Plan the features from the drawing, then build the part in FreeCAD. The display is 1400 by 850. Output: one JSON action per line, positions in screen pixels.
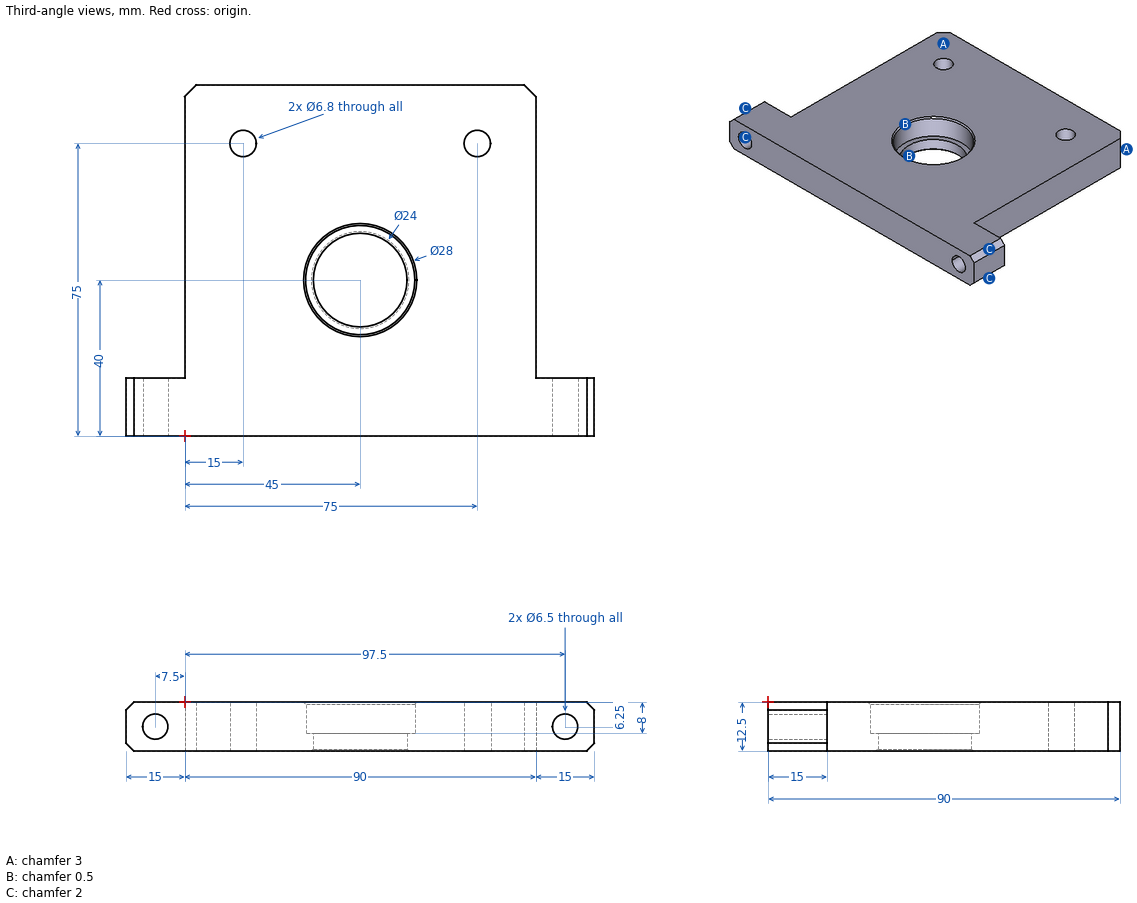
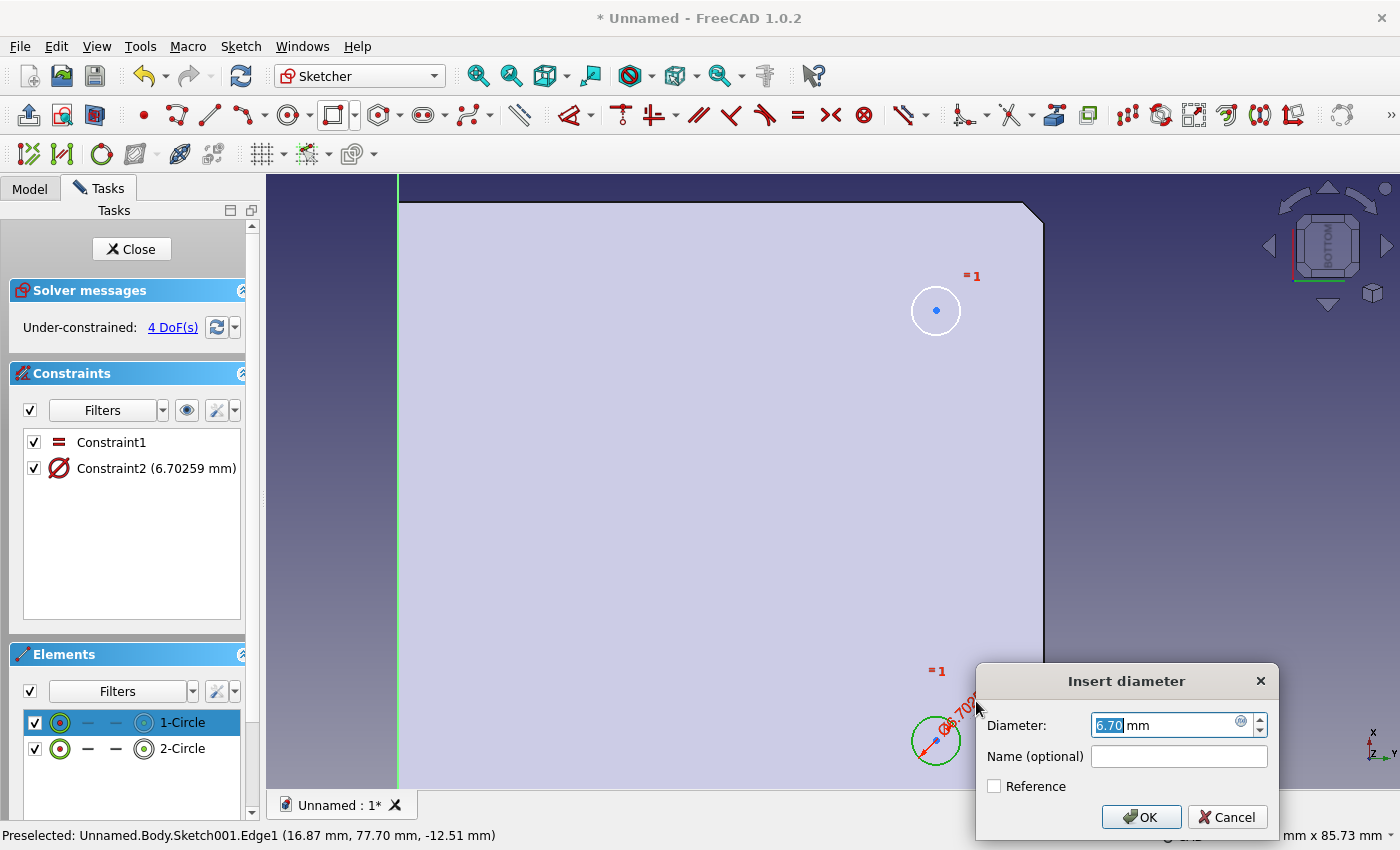
{"action": "type", "text": "6.8"}
{"action": "key", "text": "Return"}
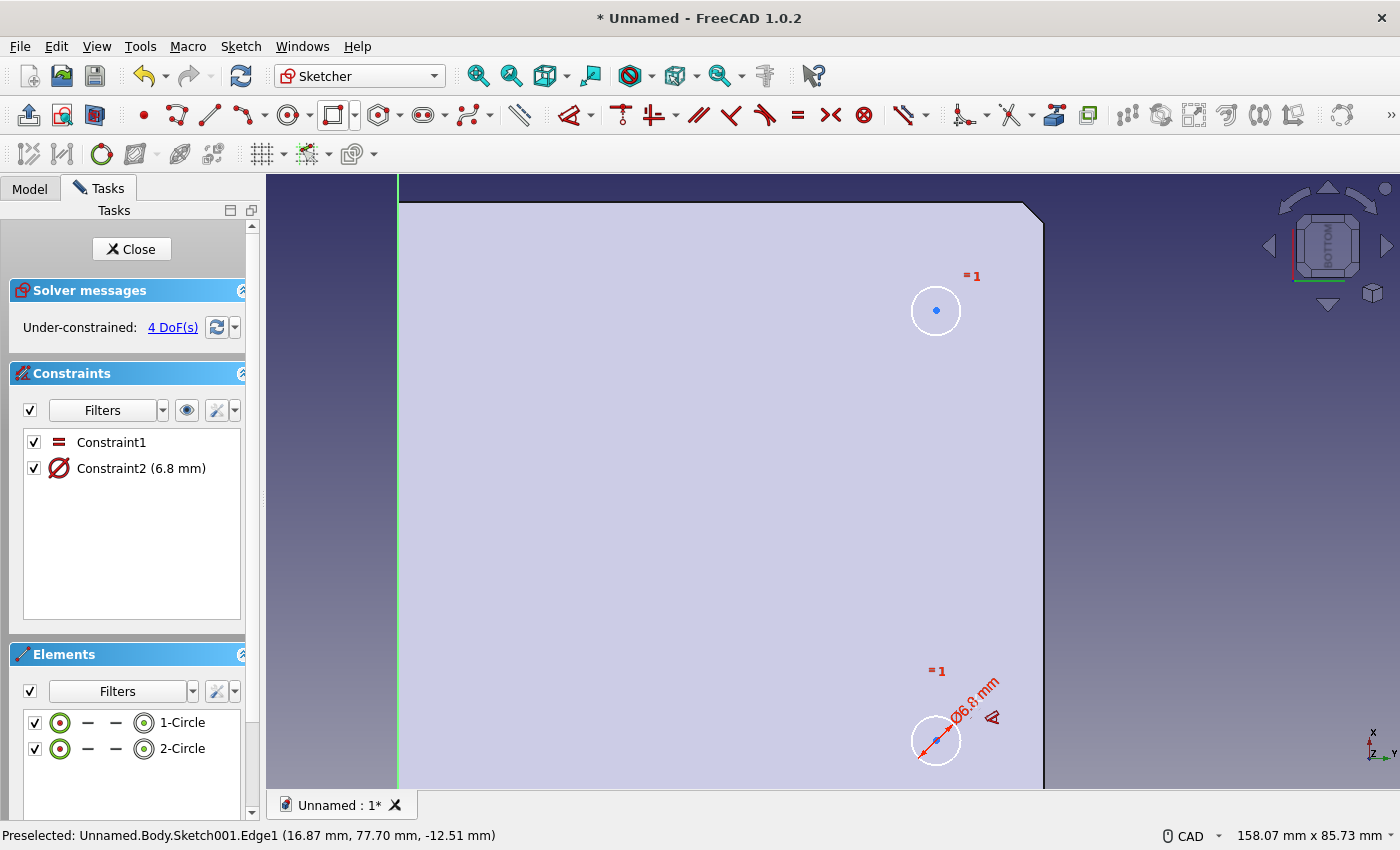
{"action": "left_click", "coordinate": [936, 741]}
{"action": "left_click", "coordinate": [667, 707]}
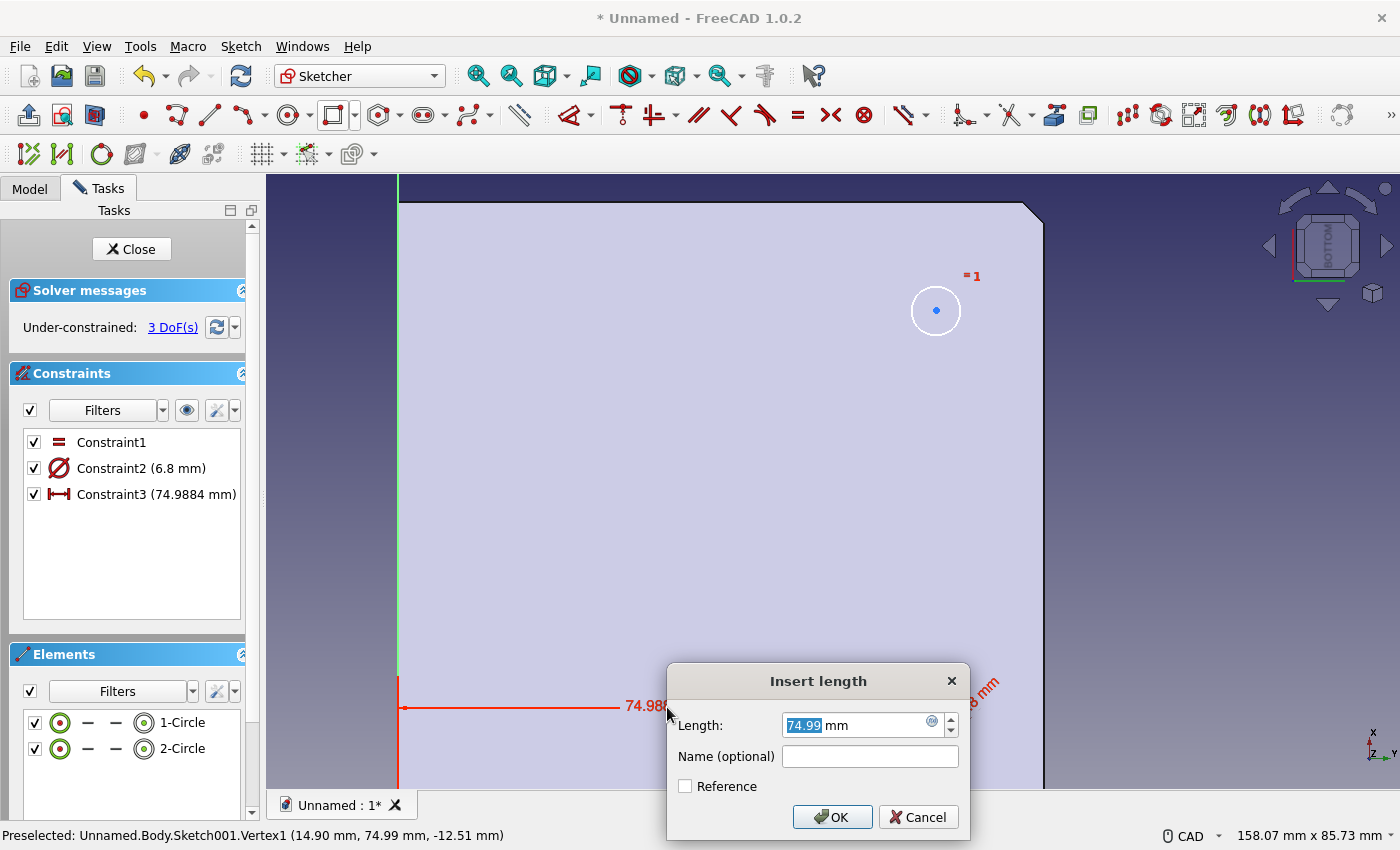
{"action": "type", "text": "75"}
{"action": "key", "text": "Return"}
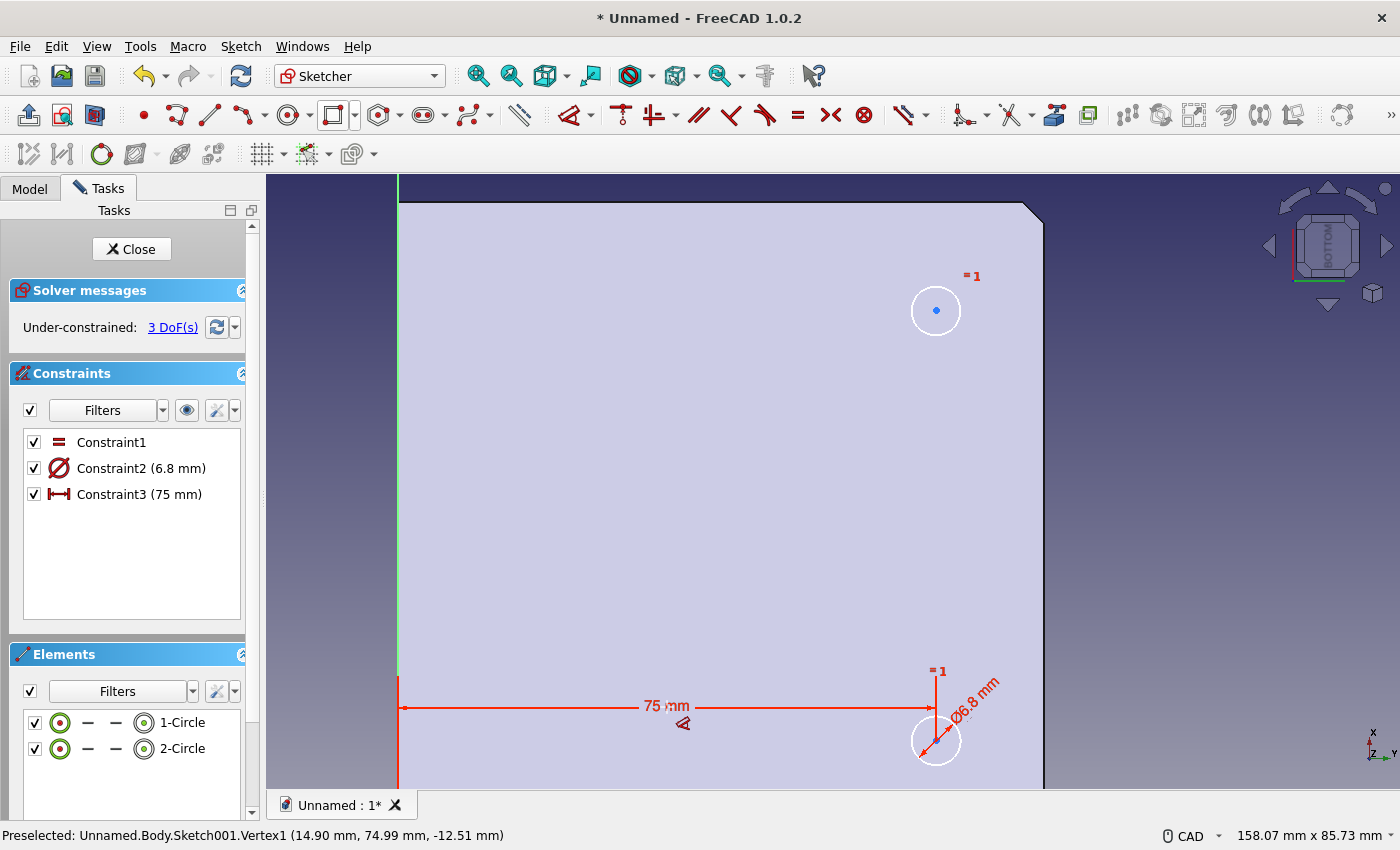
{"action": "left_click", "coordinate": [936, 741]}
{"action": "left_click", "coordinate": [364, 751]}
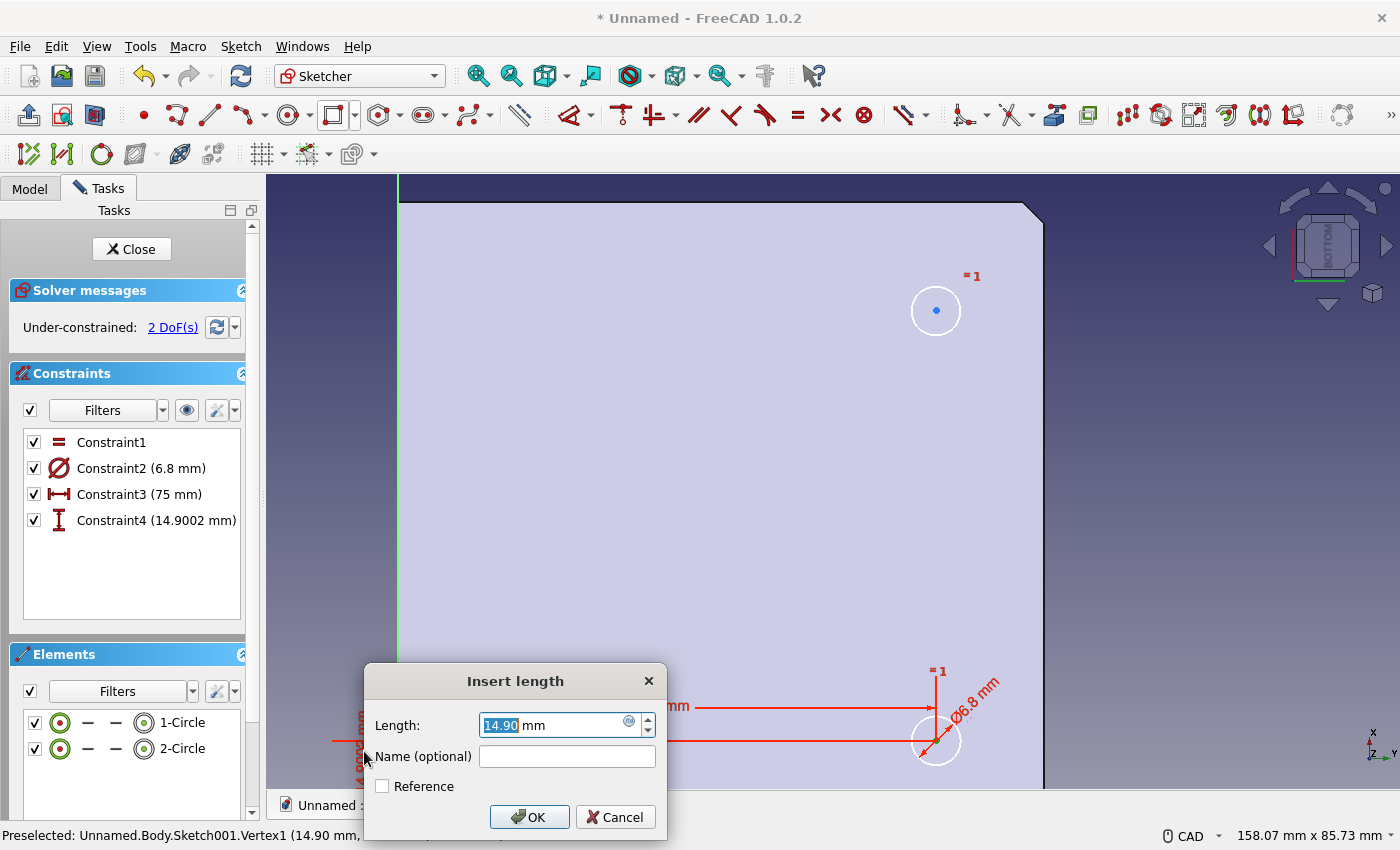
{"action": "type", "text": "15"}
{"action": "key", "text": "Return"}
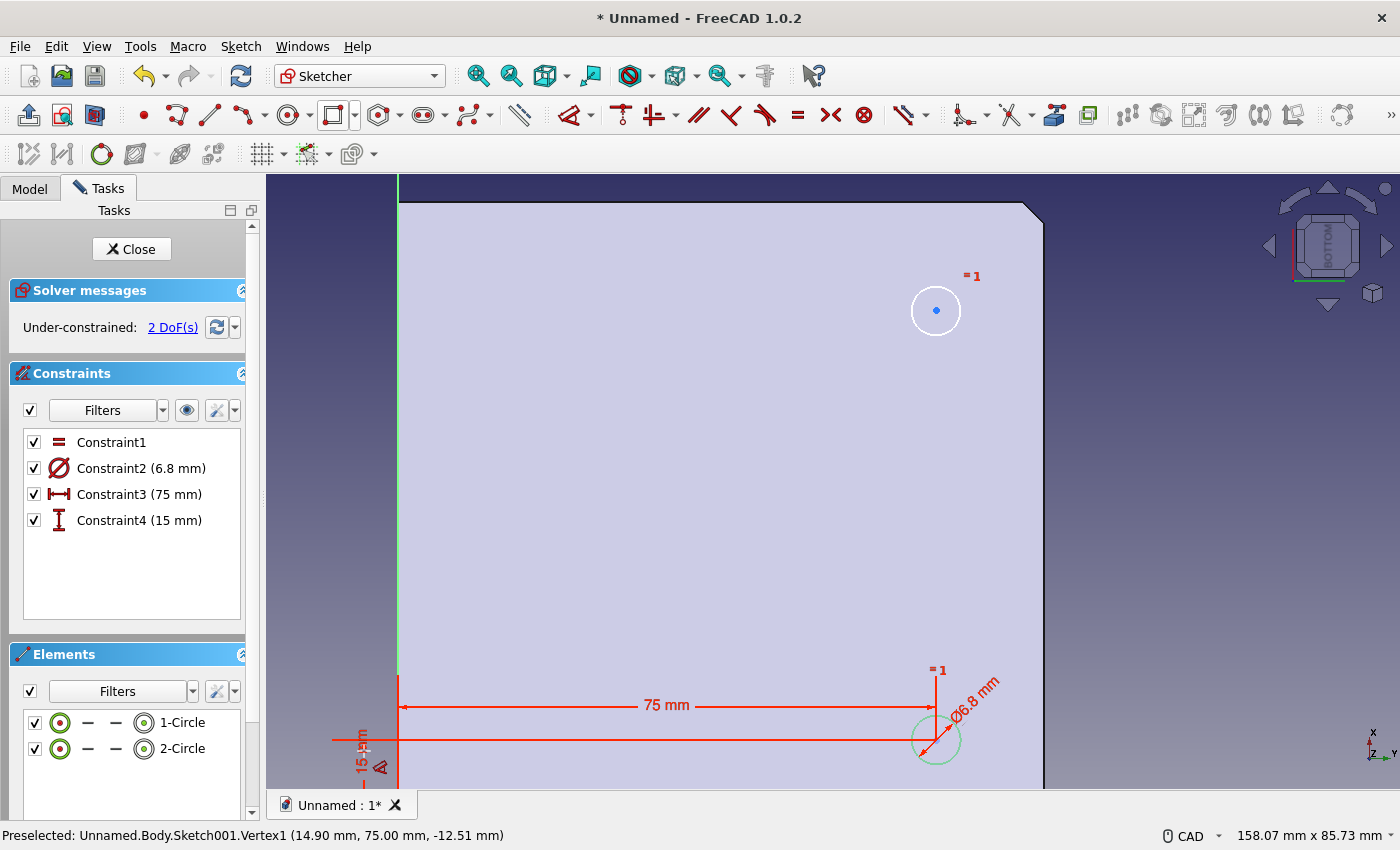
{"action": "left_click", "coordinate": [936, 311]}
{"action": "left_click", "coordinate": [667, 277]}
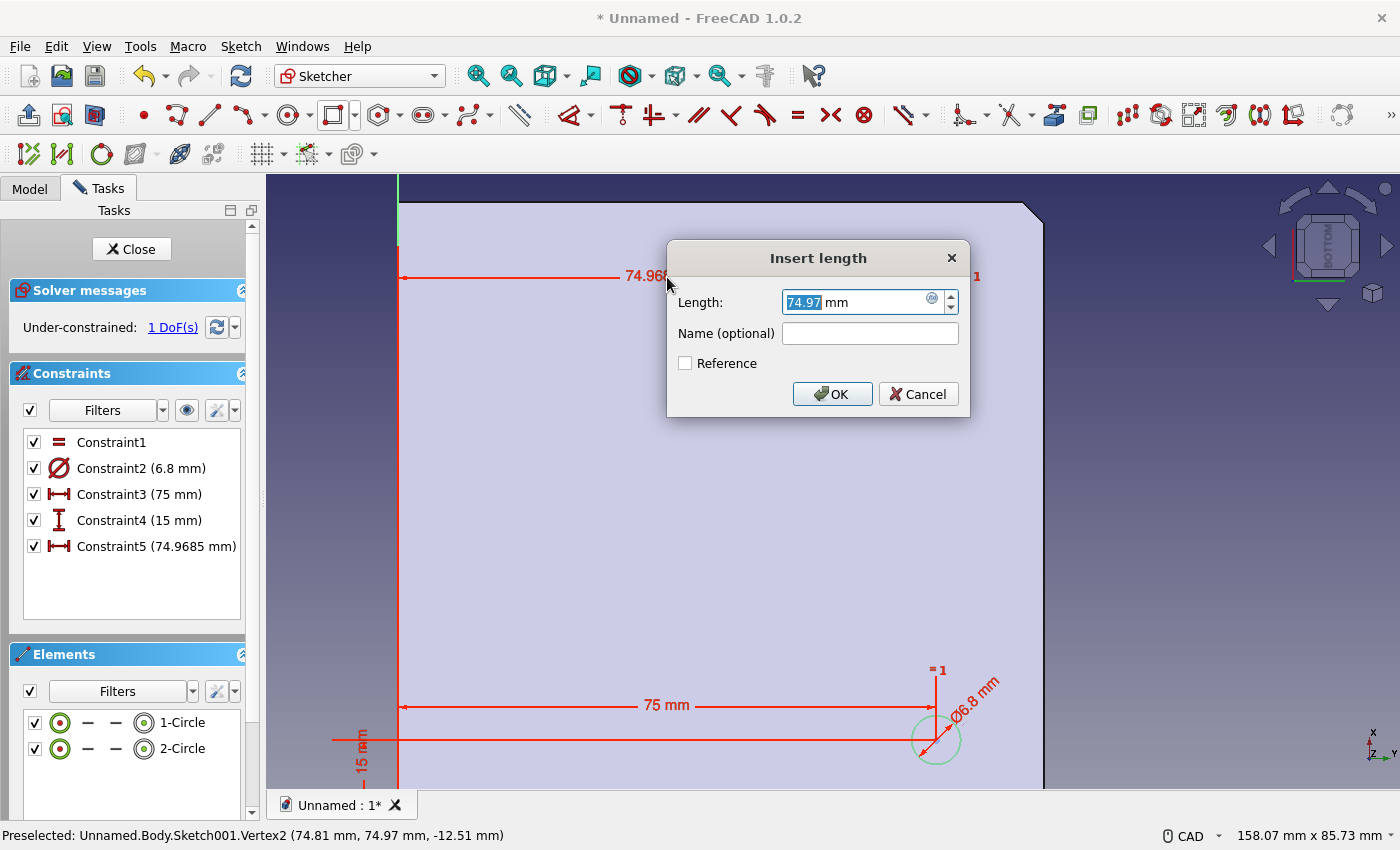
{"action": "type", "text": "75"}
{"action": "key", "text": "Return"}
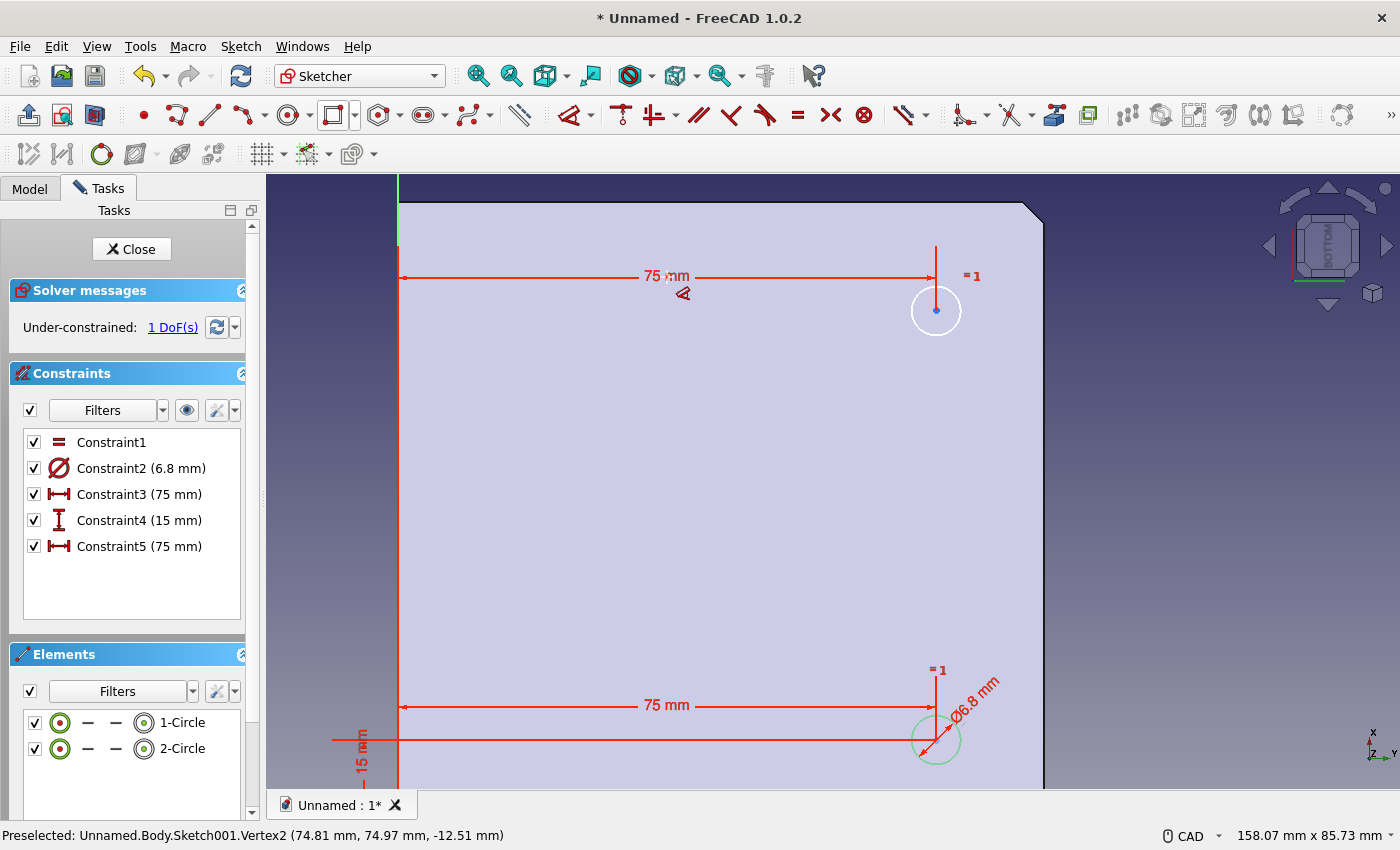
{"action": "left_click", "coordinate": [936, 311]}
{"action": "left_click", "coordinate": [364, 536]}